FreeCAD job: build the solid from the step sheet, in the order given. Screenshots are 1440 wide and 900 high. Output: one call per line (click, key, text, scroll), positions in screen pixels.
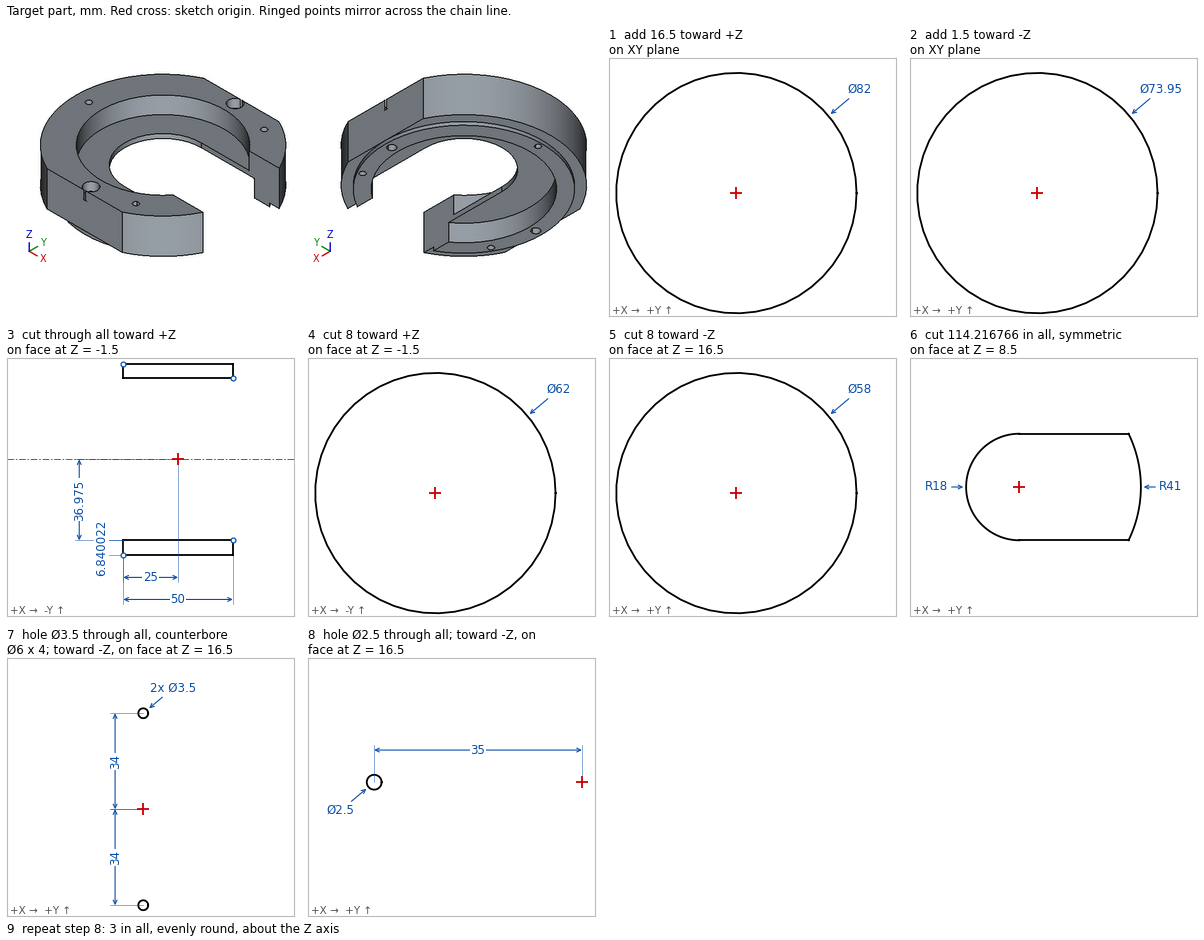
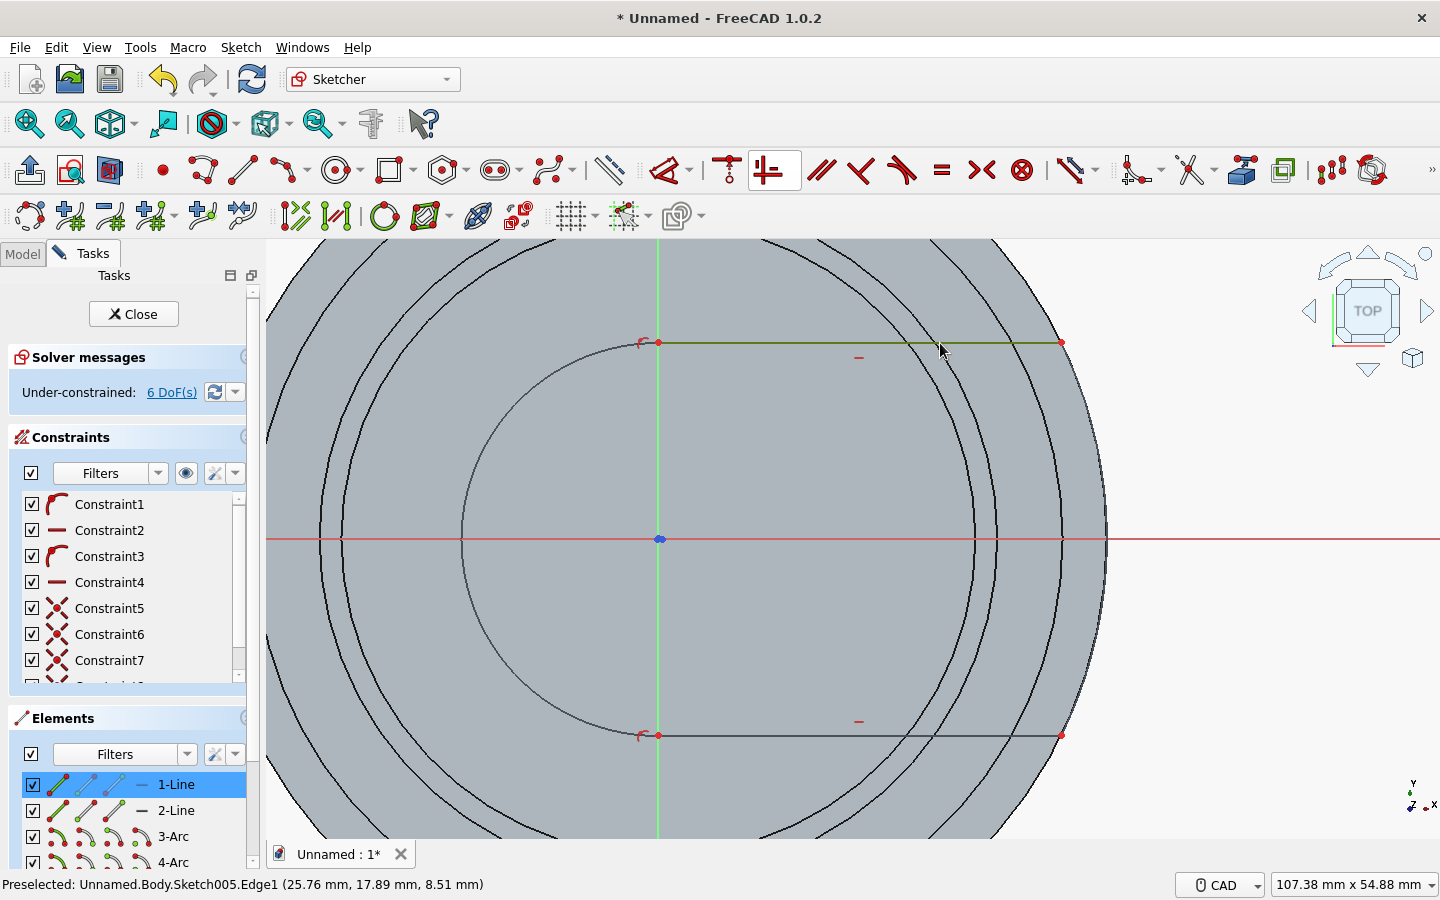
click(499, 424)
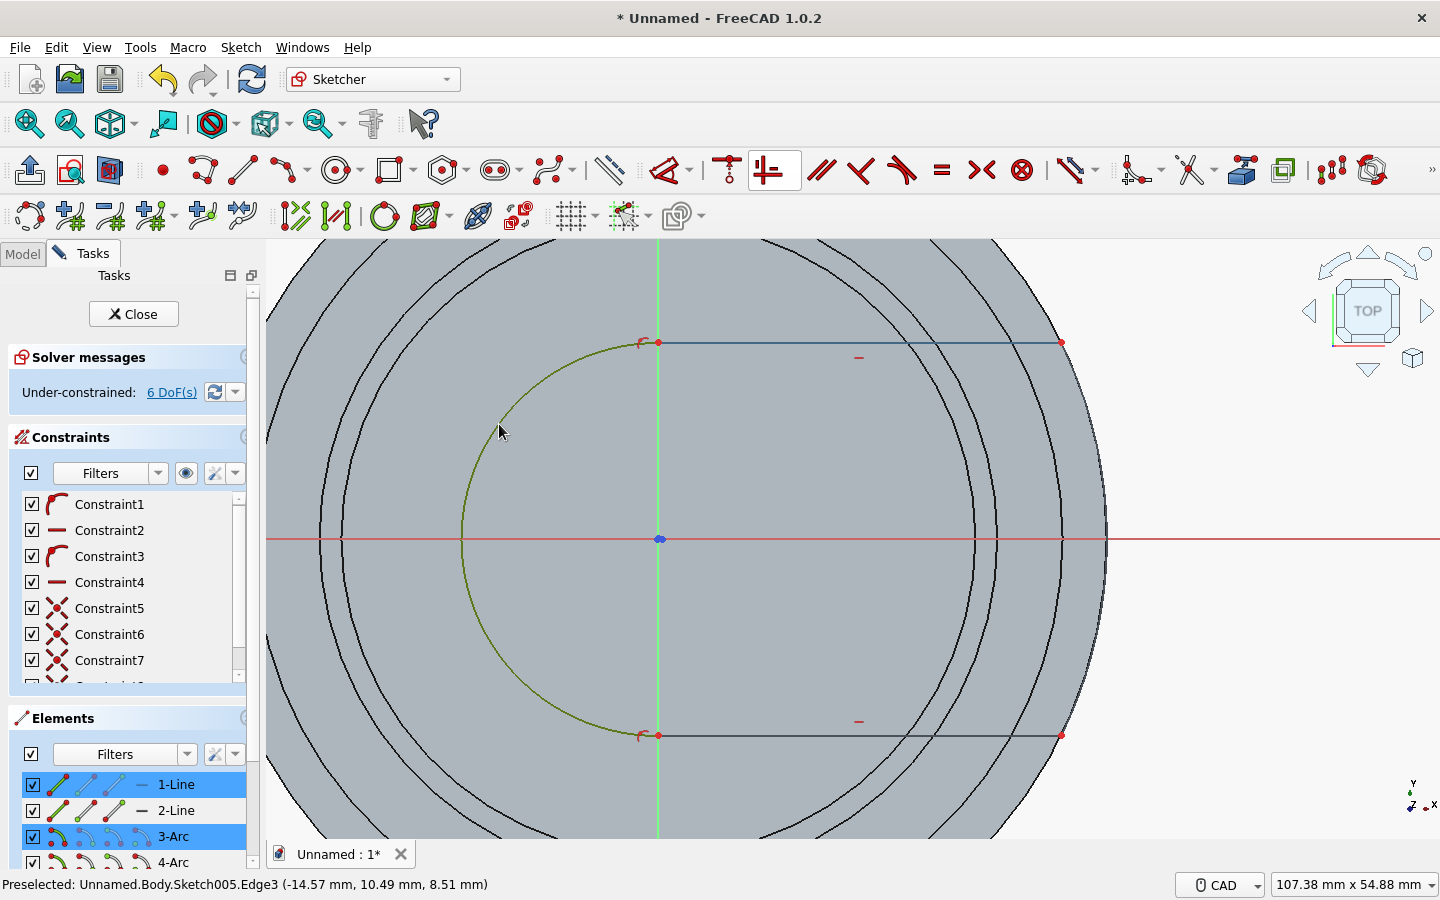
key(t)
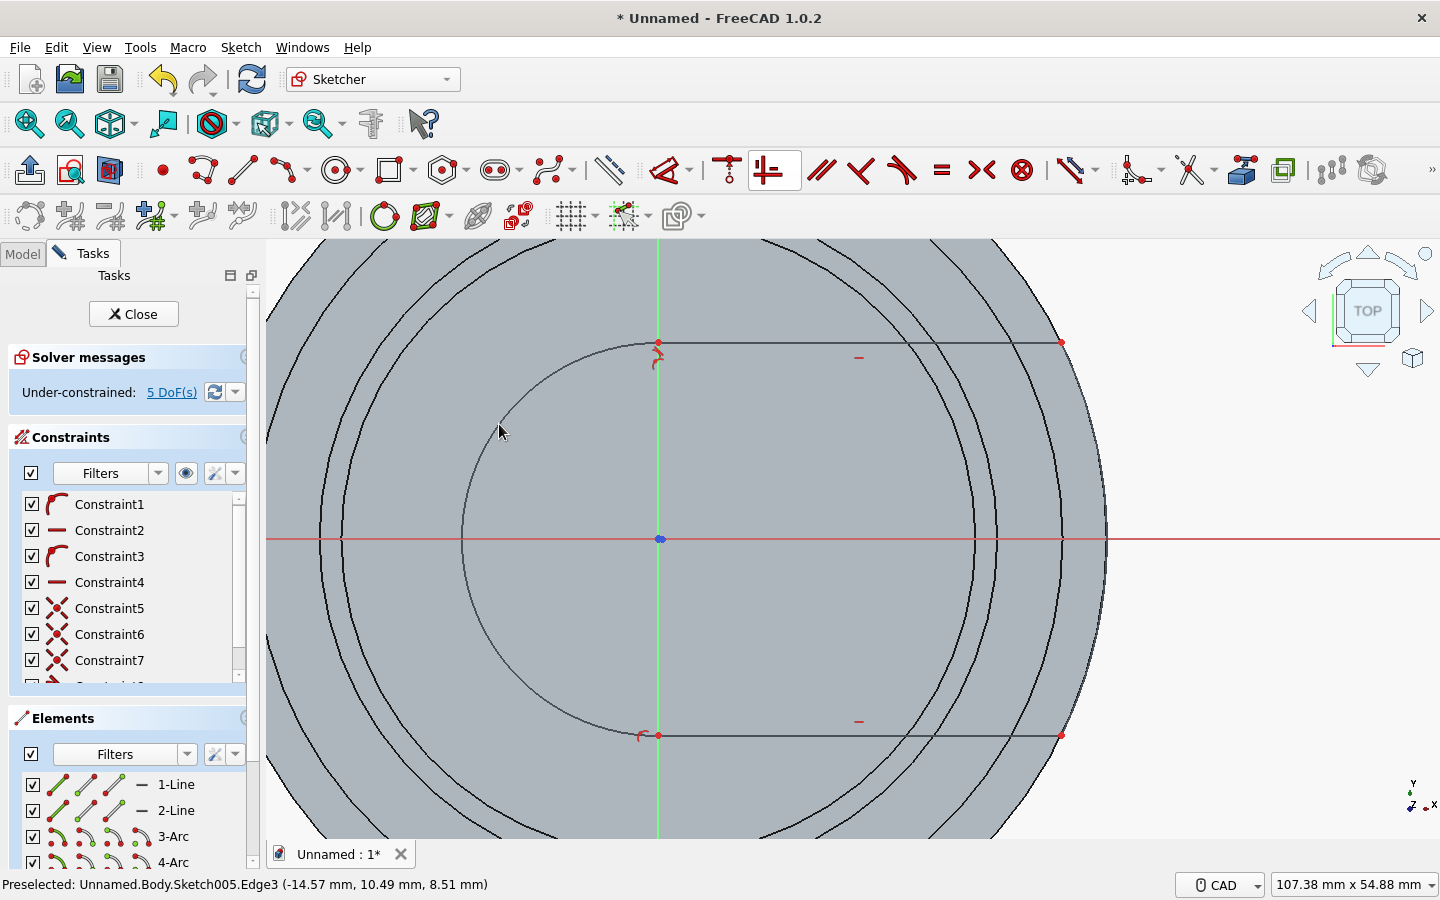
click(499, 424)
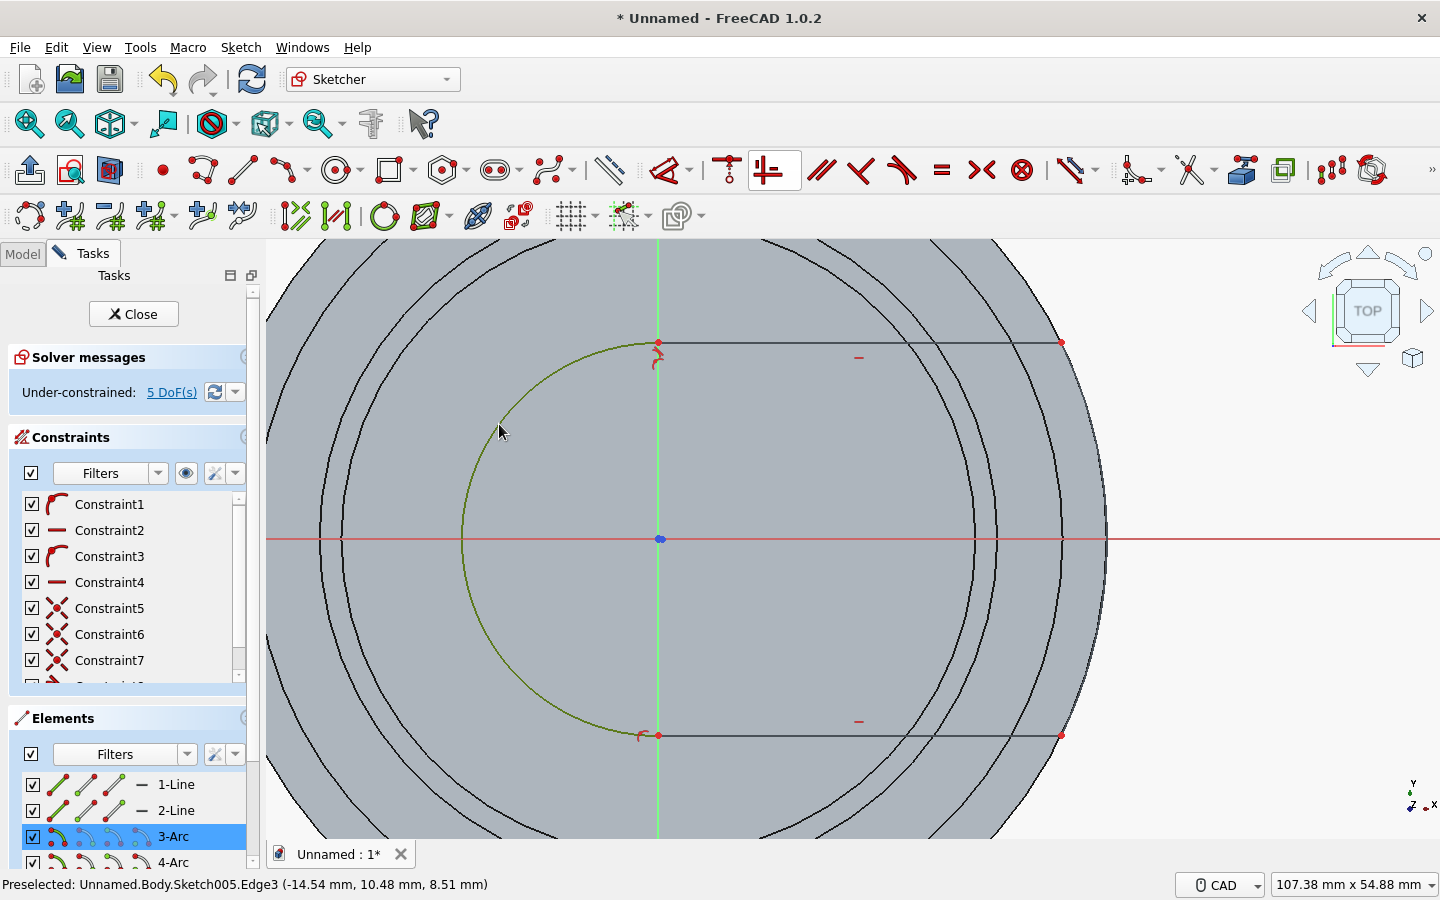
click(1099, 620)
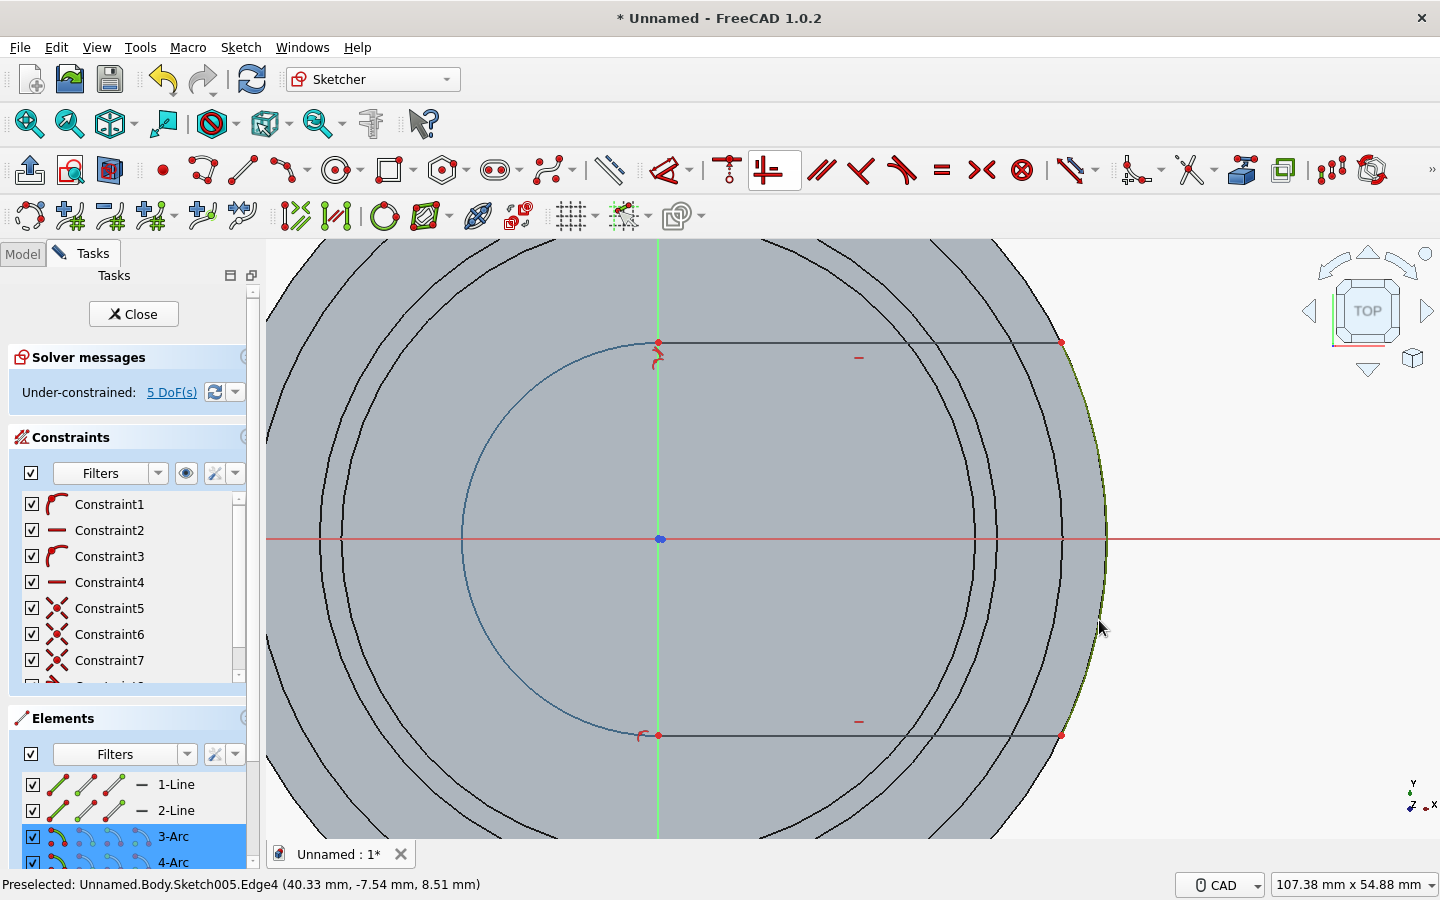
click(728, 170)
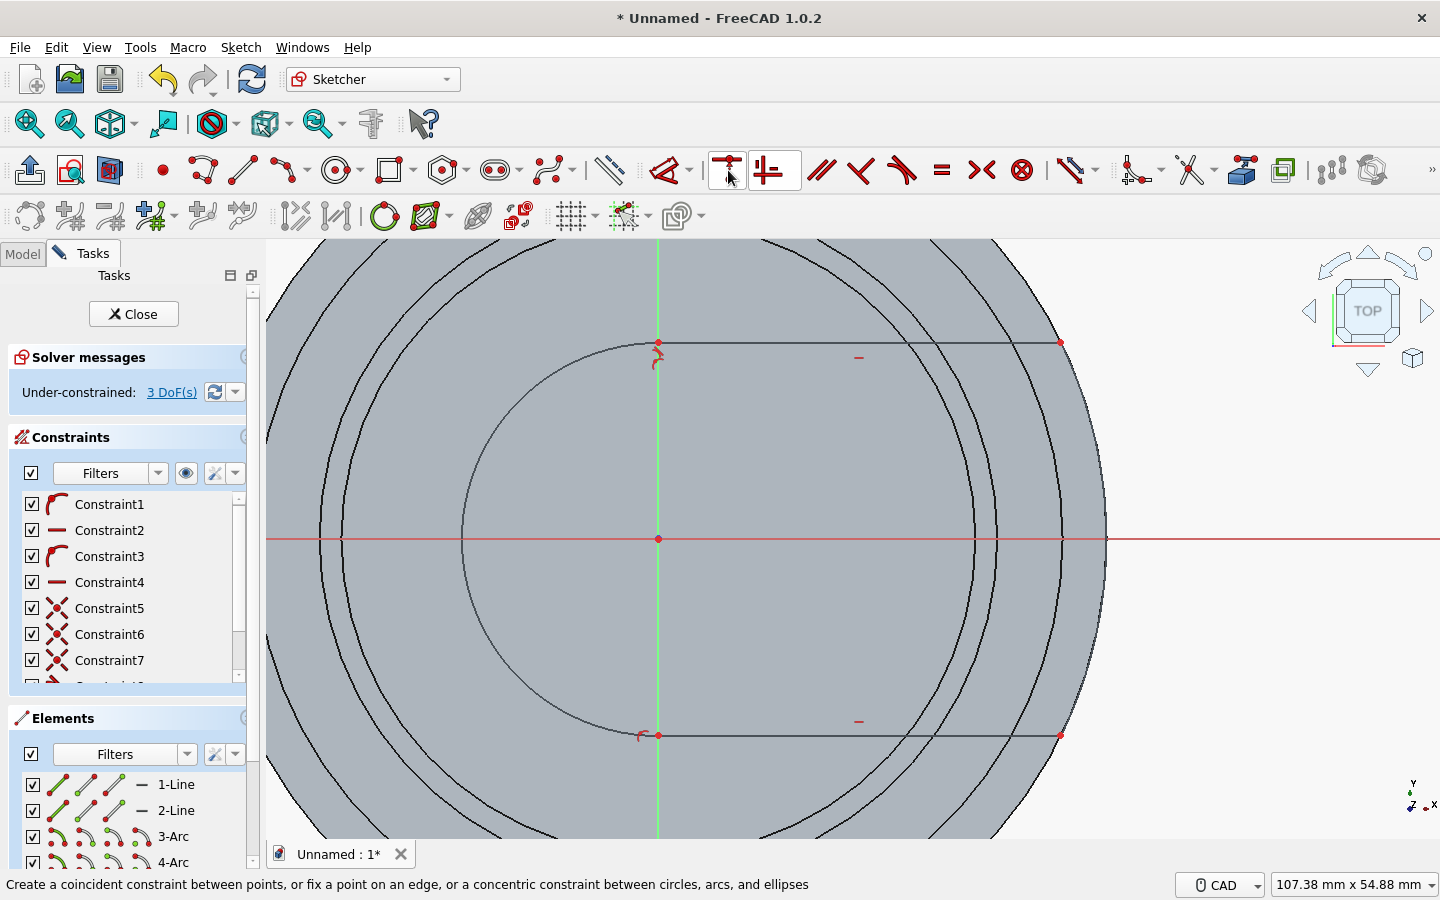
click(658, 540)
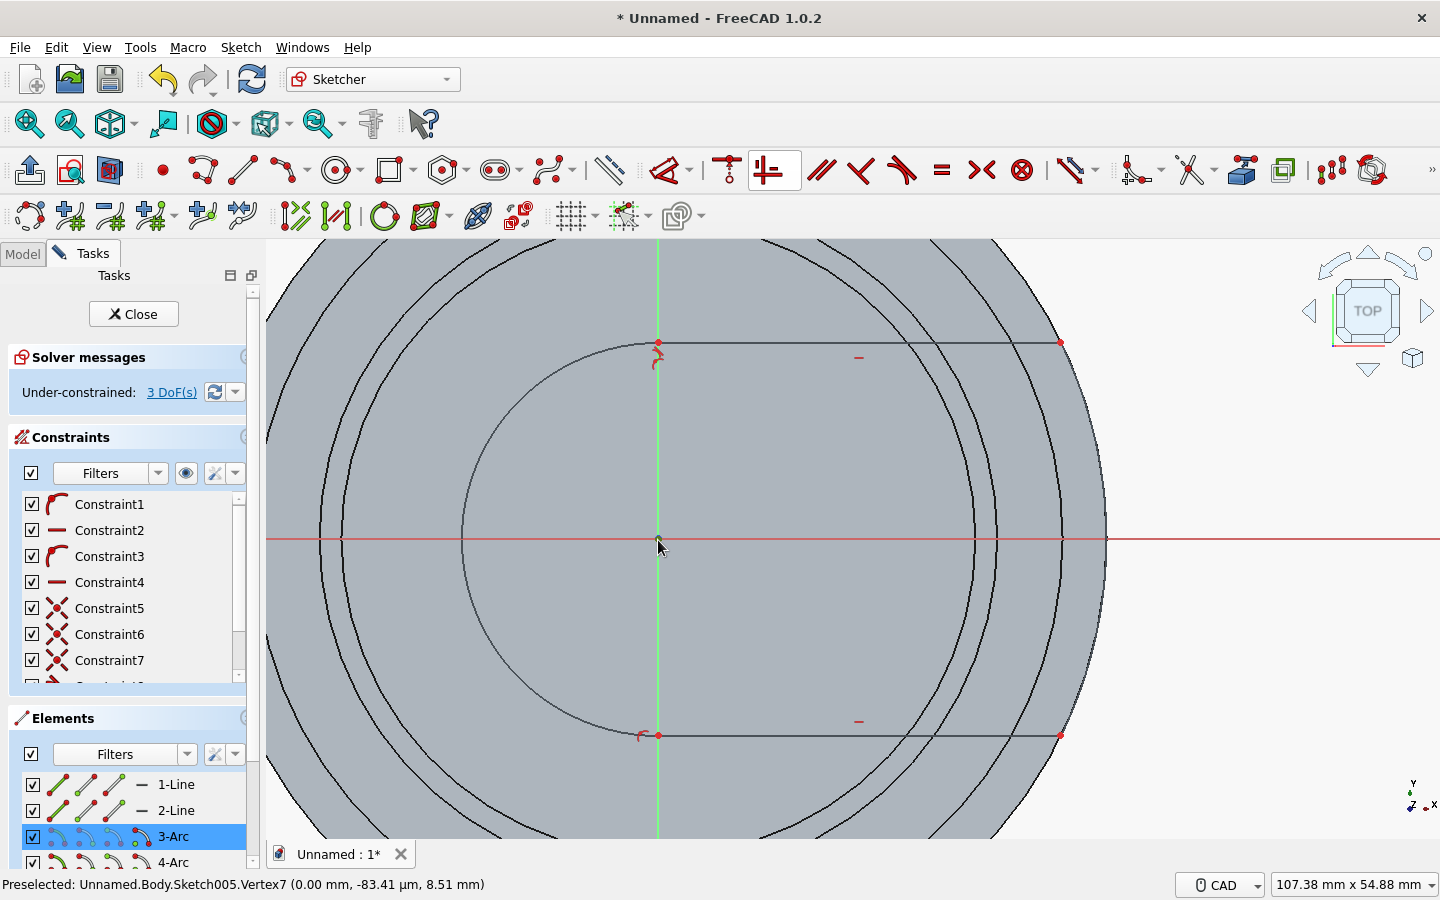
click(364, 539)